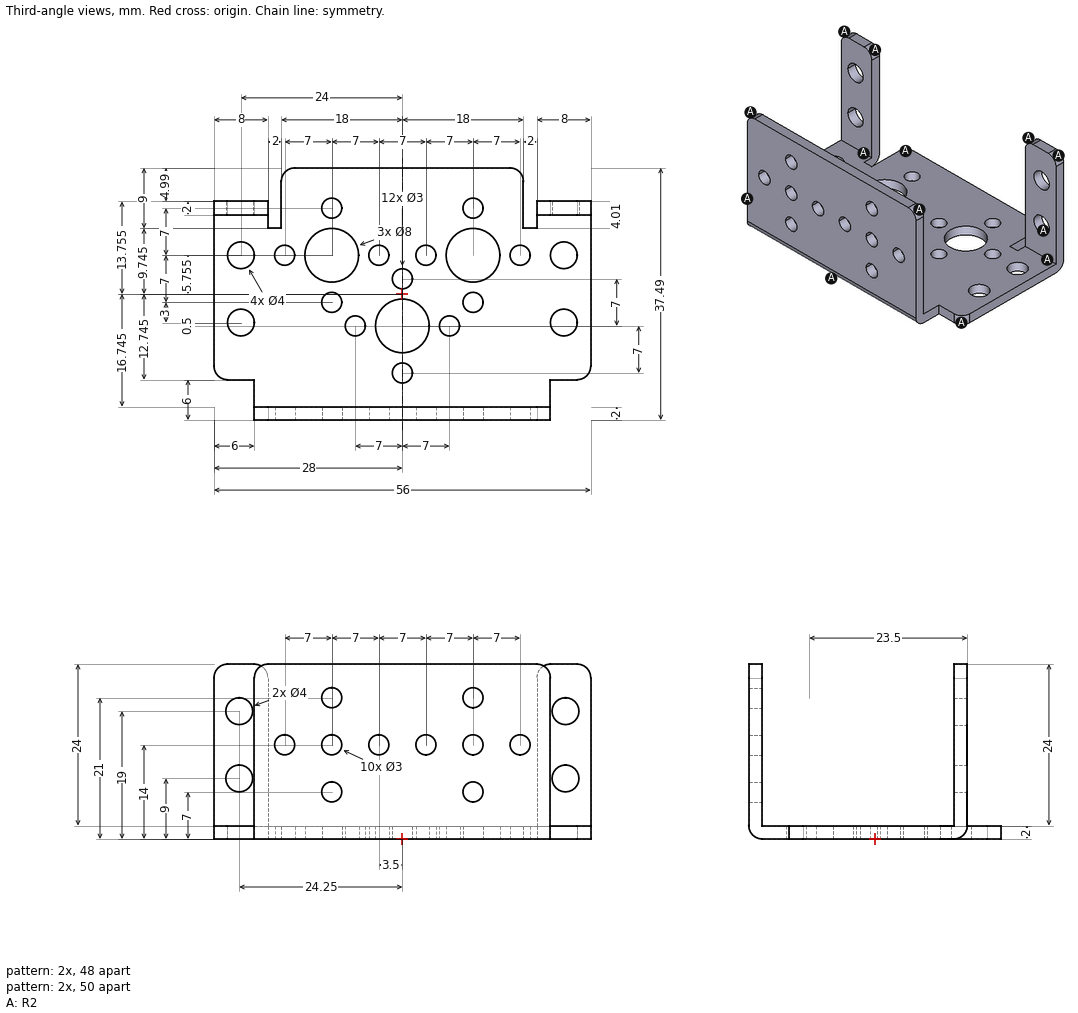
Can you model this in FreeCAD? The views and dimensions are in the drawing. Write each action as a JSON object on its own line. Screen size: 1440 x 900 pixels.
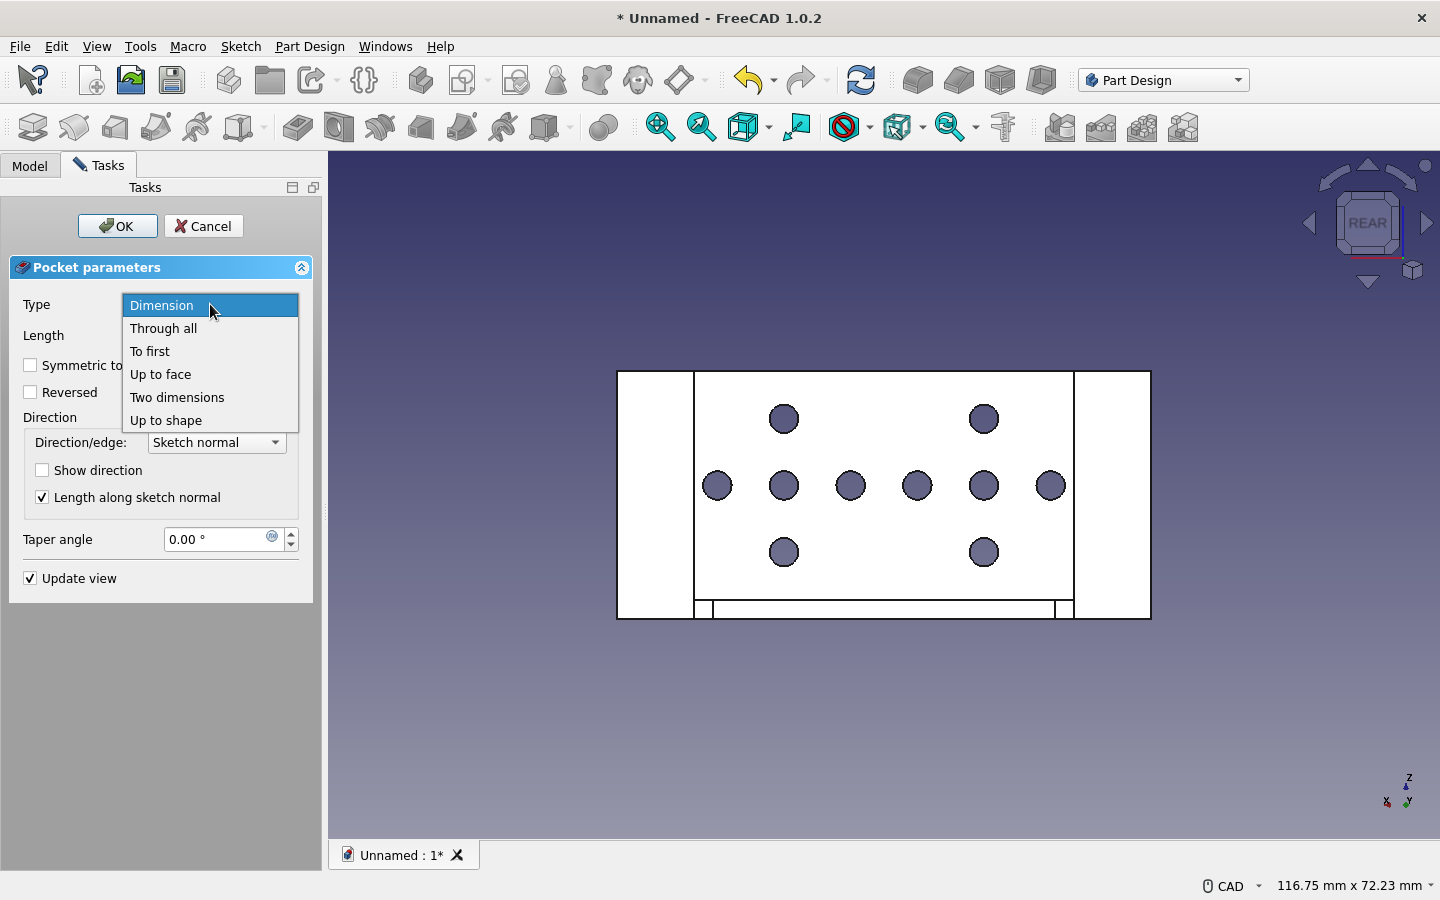
{"action": "left_click", "coordinate": [208, 328]}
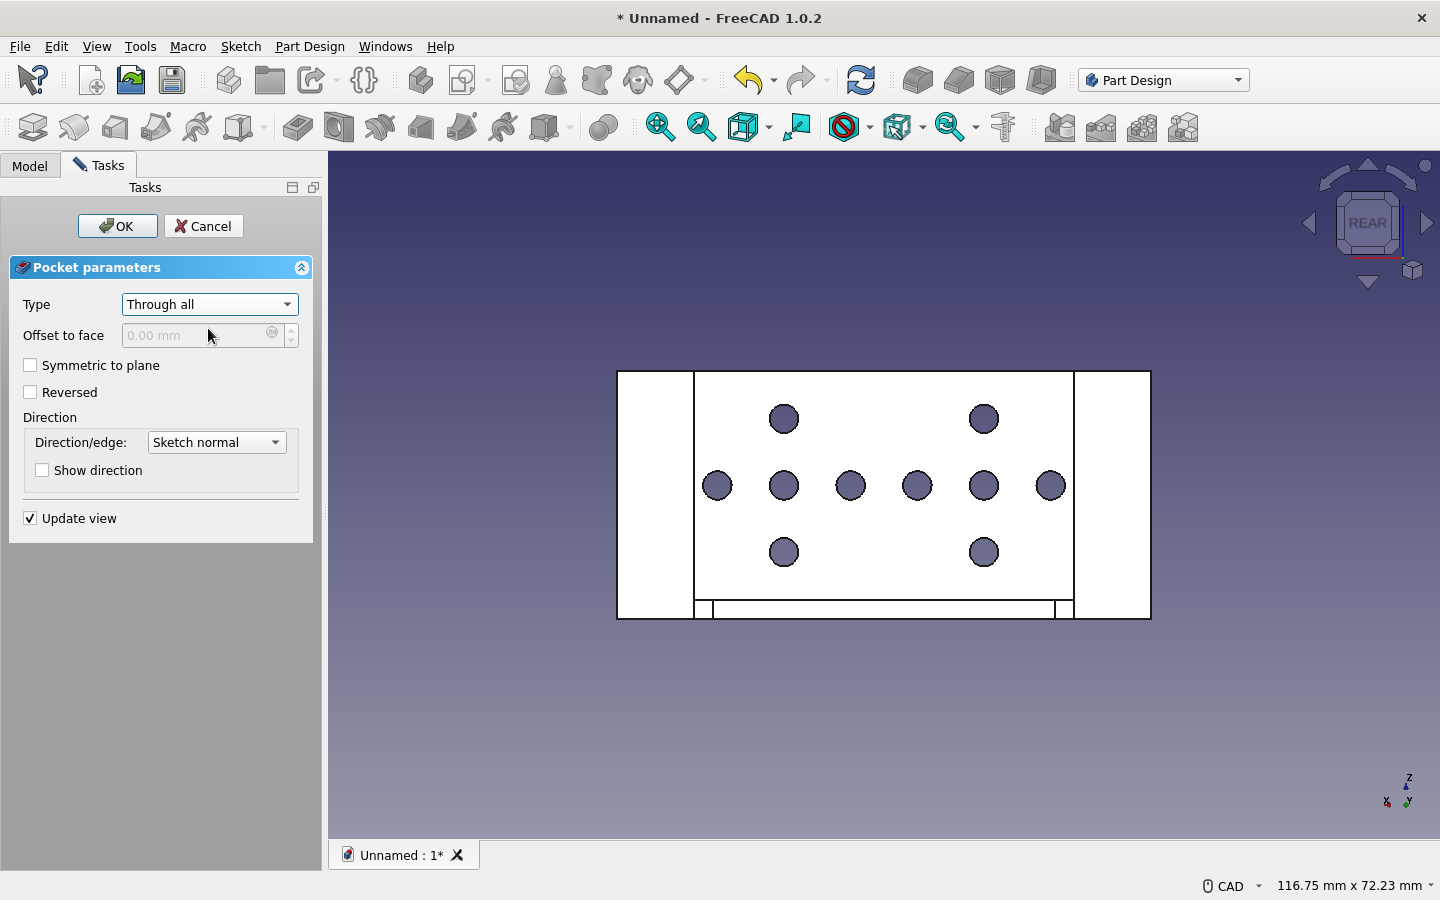
{"action": "left_click", "coordinate": [118, 226]}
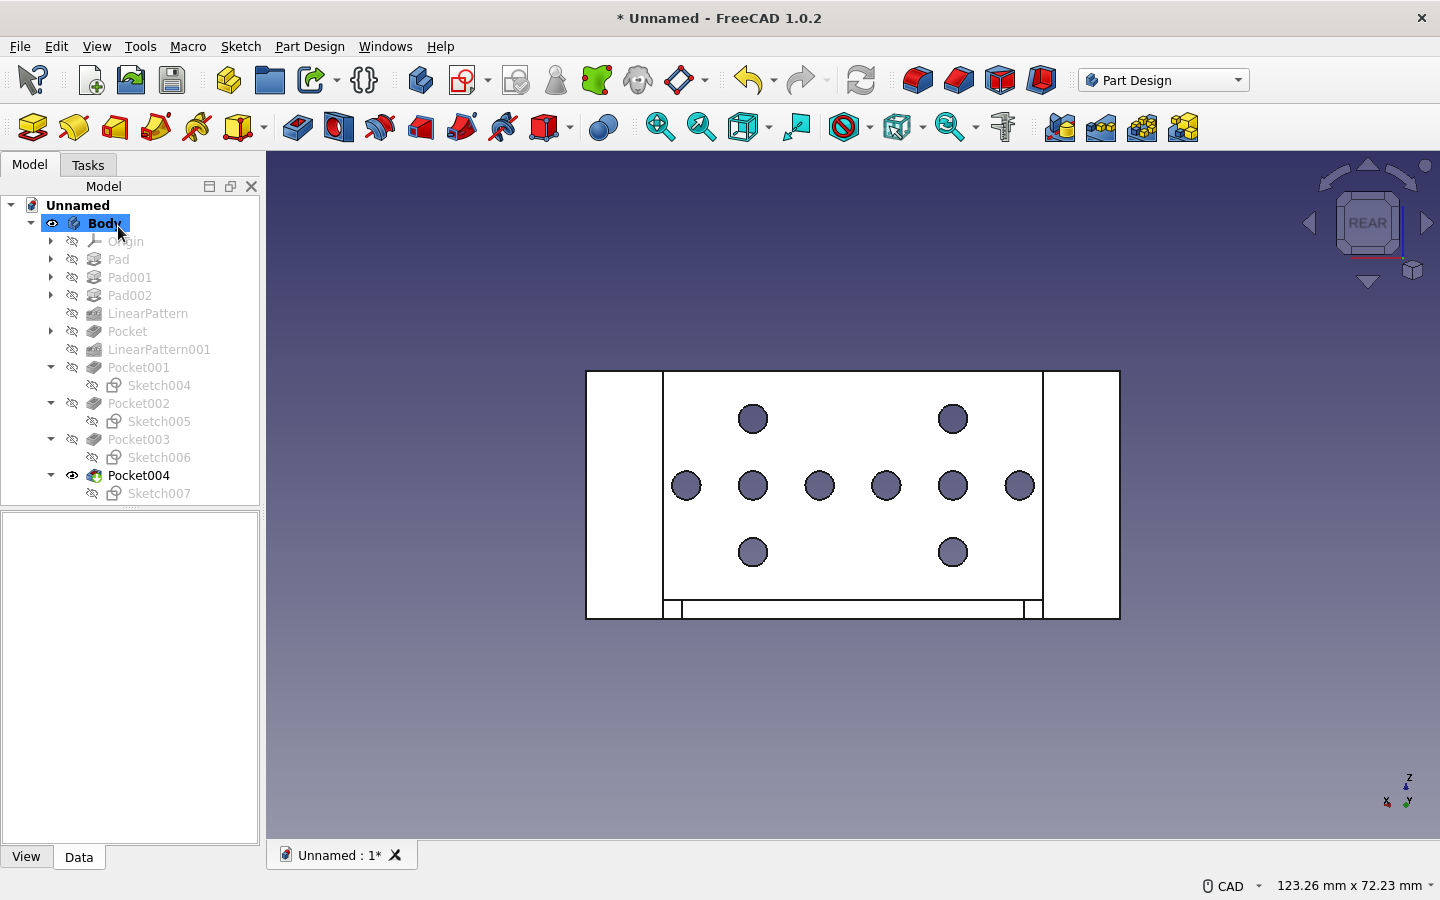
{"action": "left_click", "coordinate": [1082, 618]}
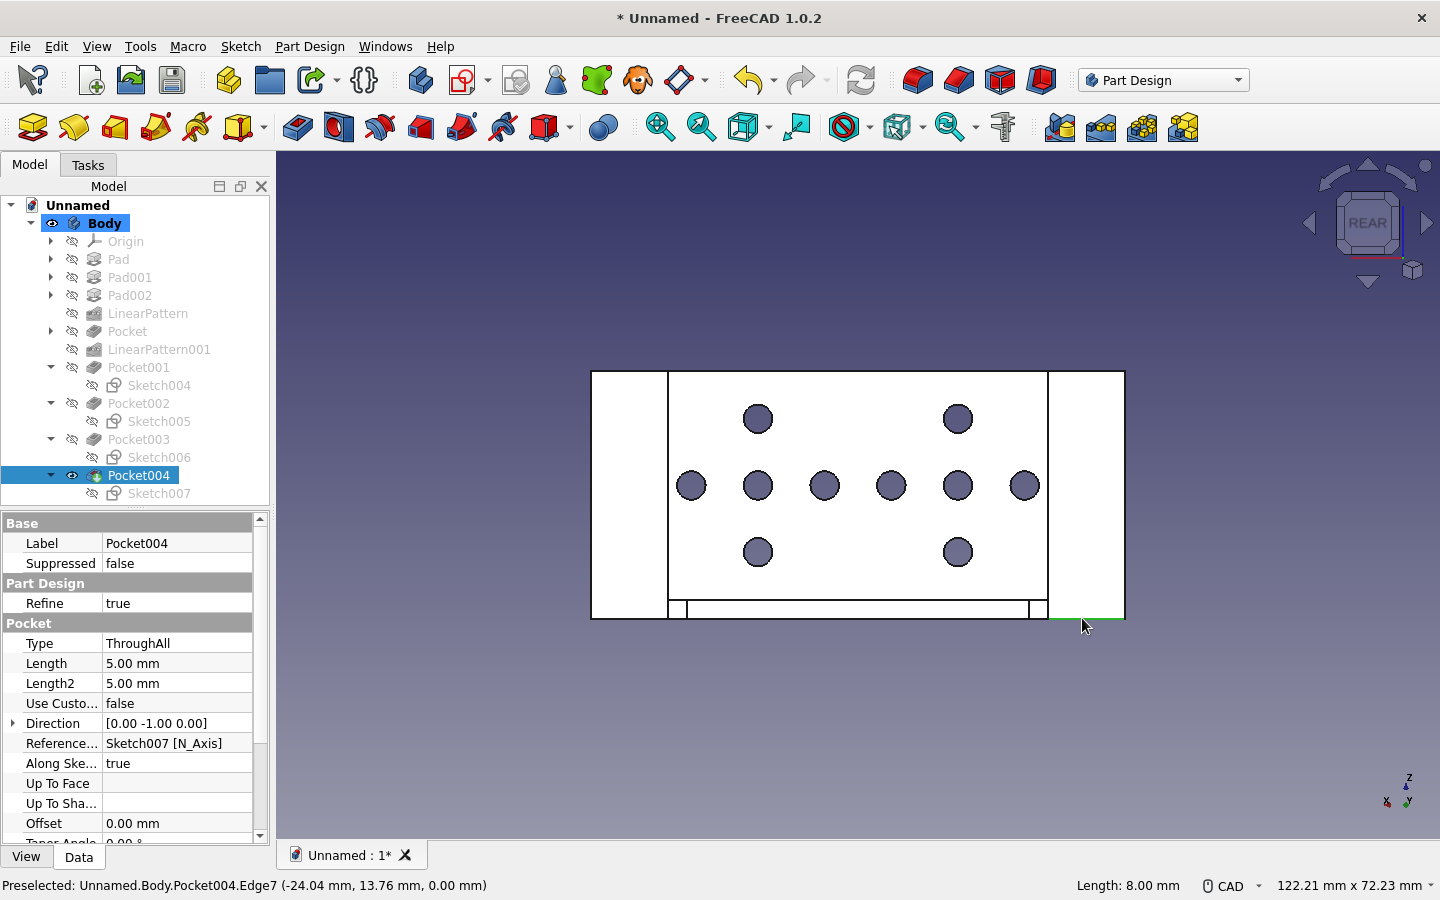
{"action": "left_click", "coordinate": [1029, 608], "text": "ctrl"}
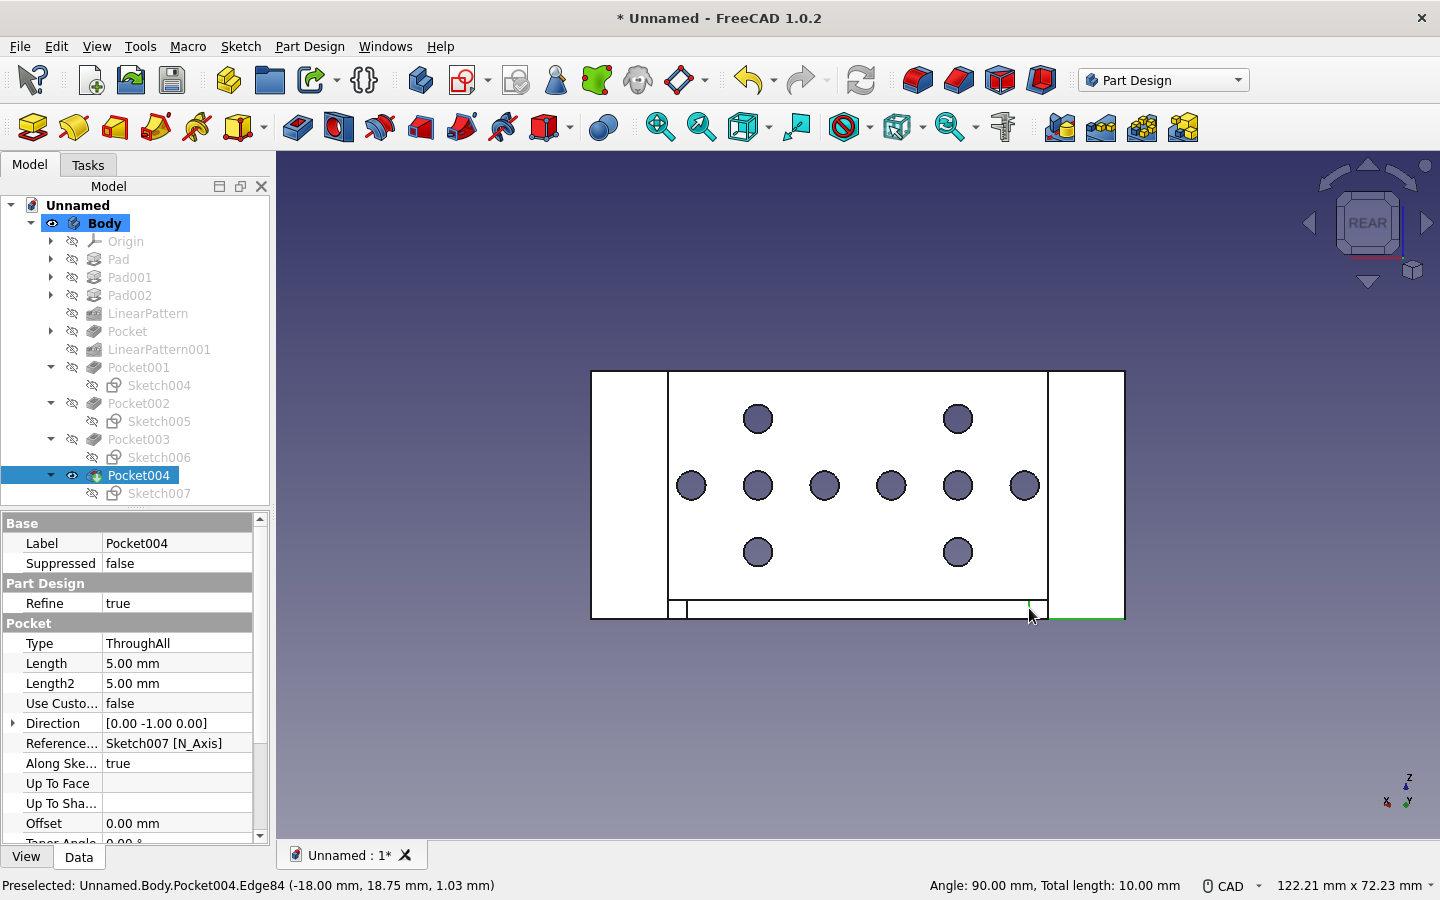
{"action": "left_click", "coordinate": [629, 618], "text": "ctrl"}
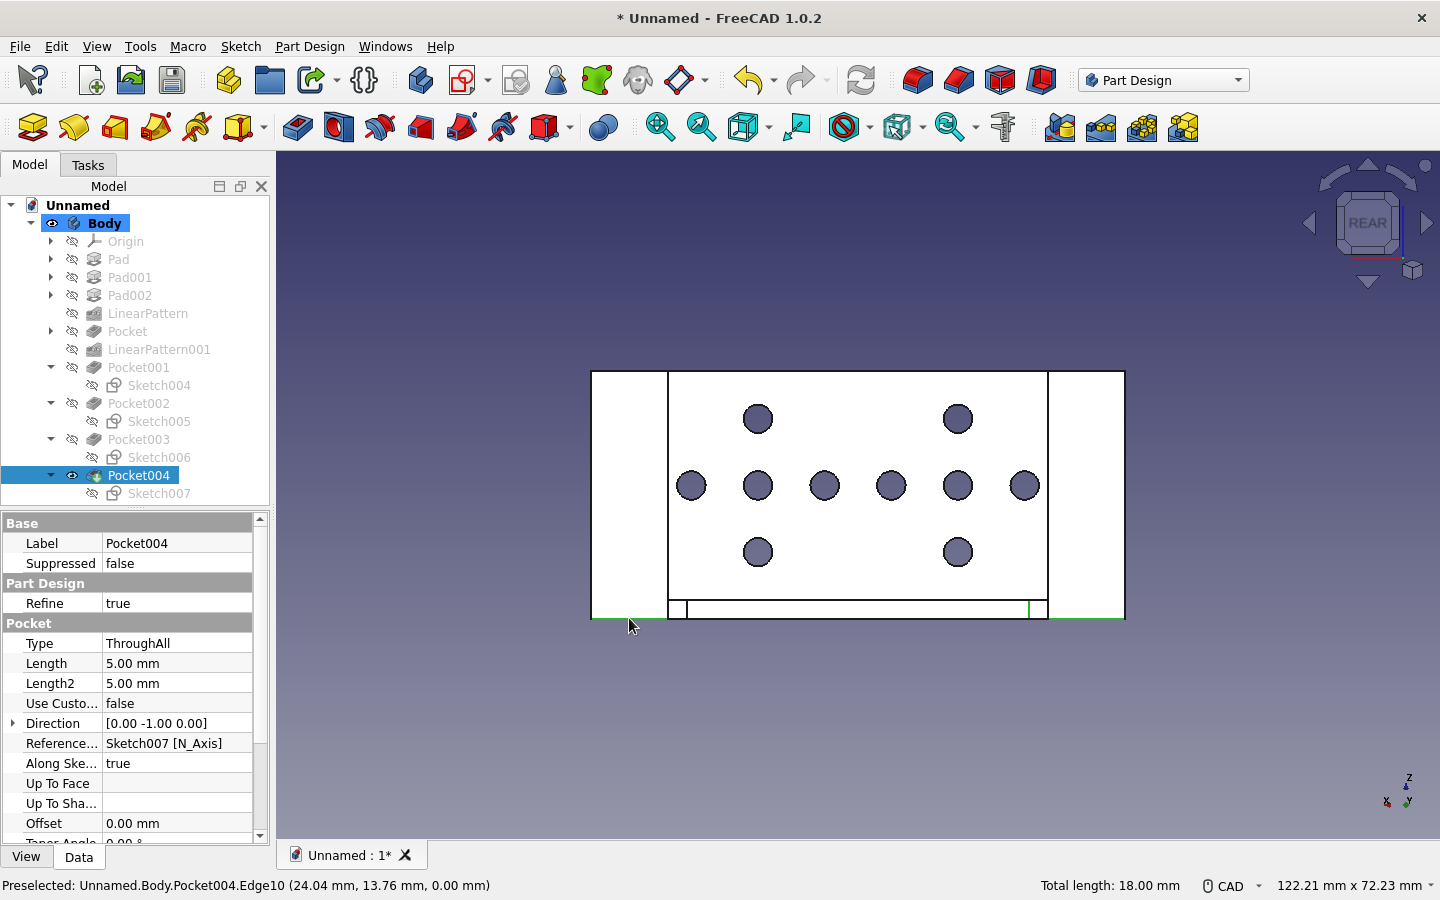
{"action": "scroll", "coordinate": [687, 608], "scroll_direction": "up", "scroll_amount": 4}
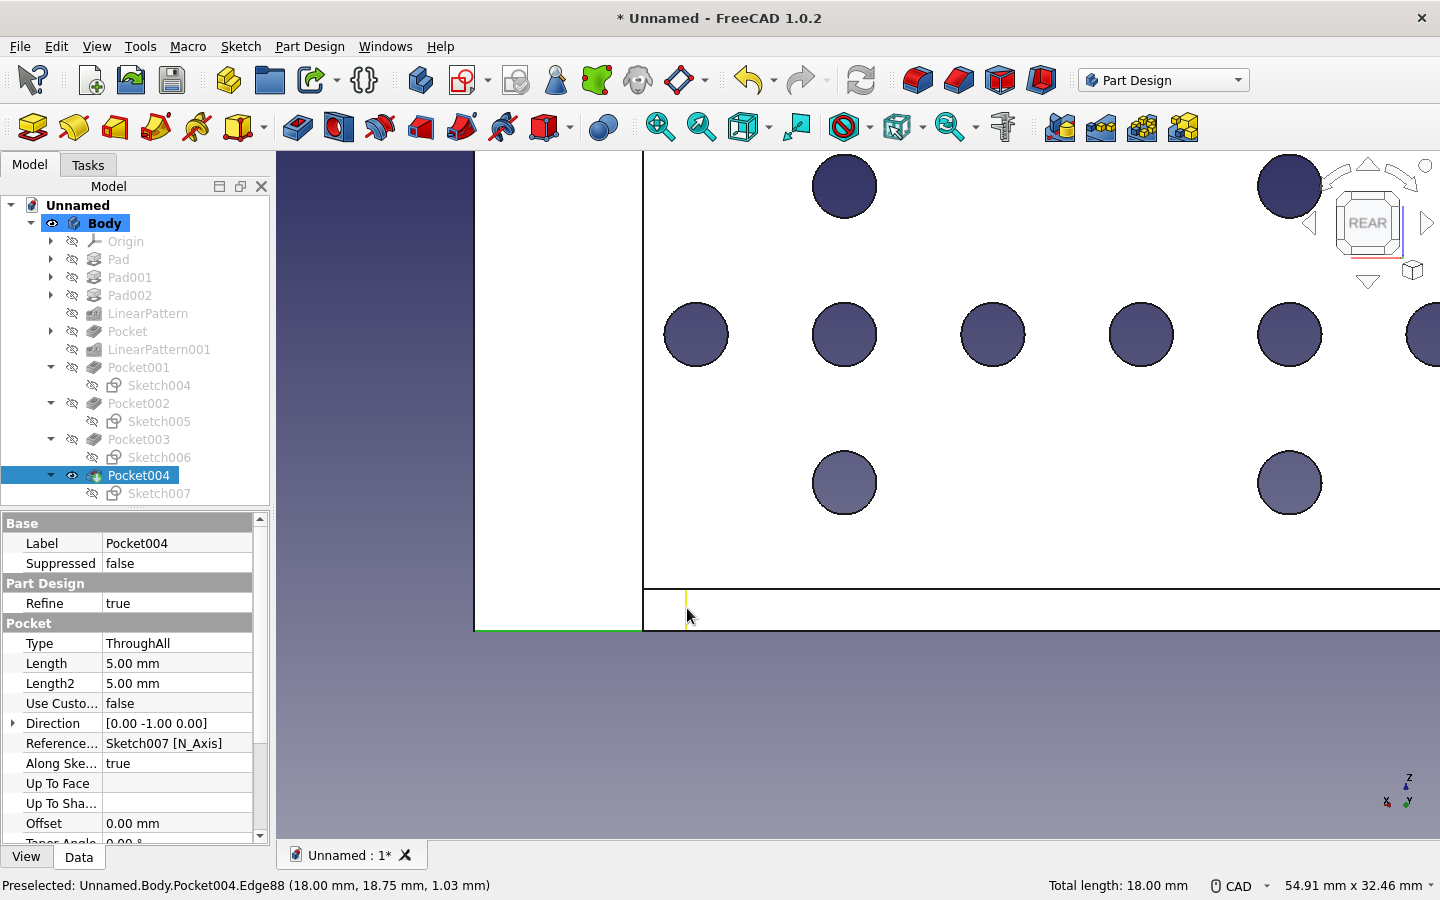
{"action": "key", "text": "v f"}